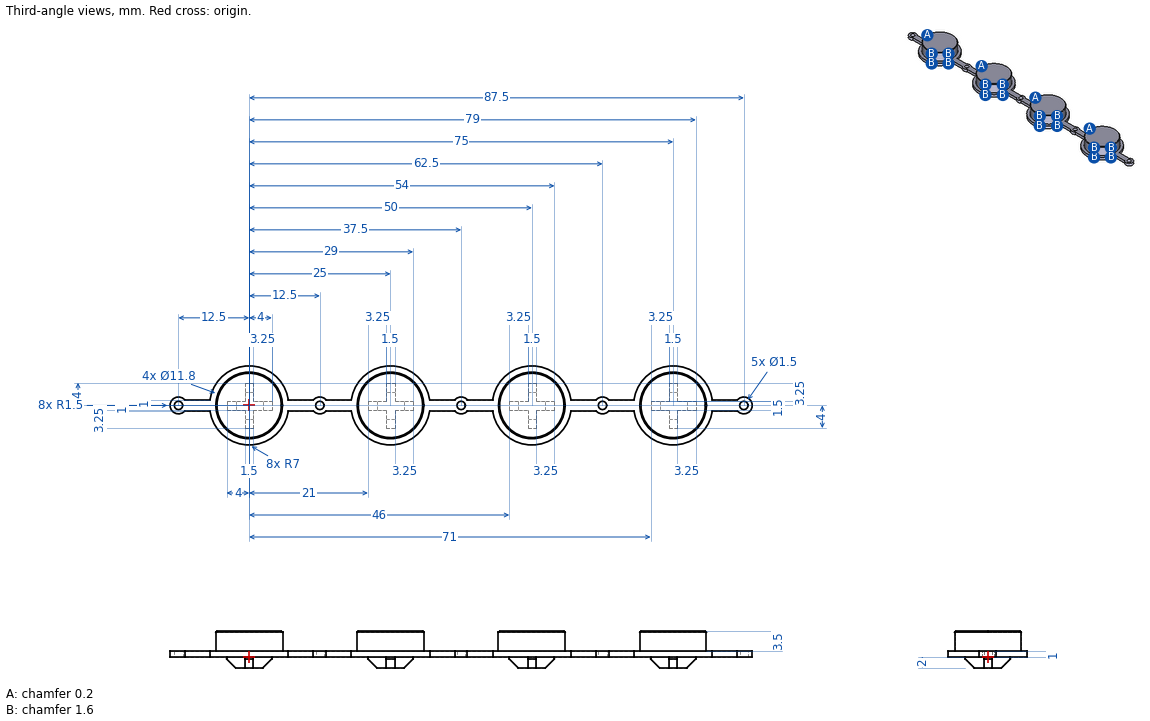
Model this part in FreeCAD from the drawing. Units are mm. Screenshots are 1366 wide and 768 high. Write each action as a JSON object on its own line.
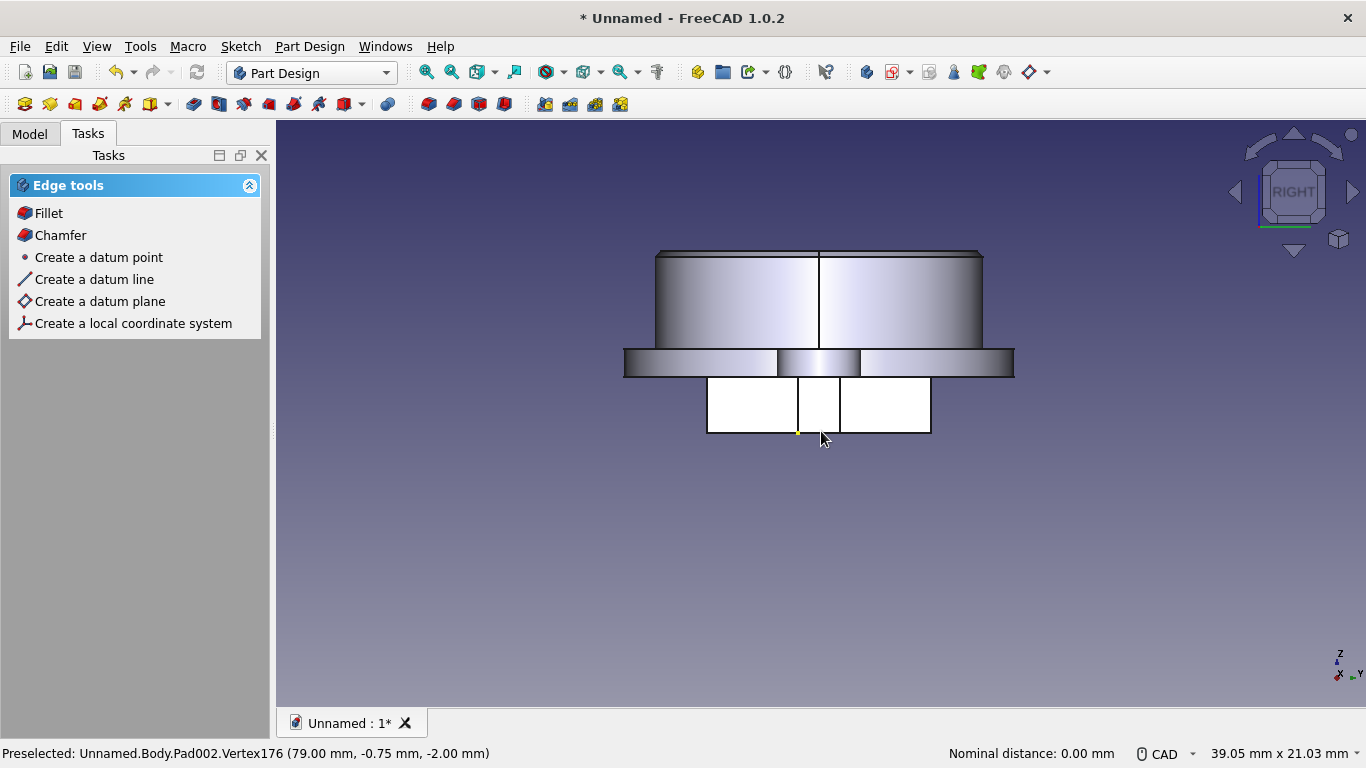
{"action": "left_click", "coordinate": [819, 432], "text": "ctrl"}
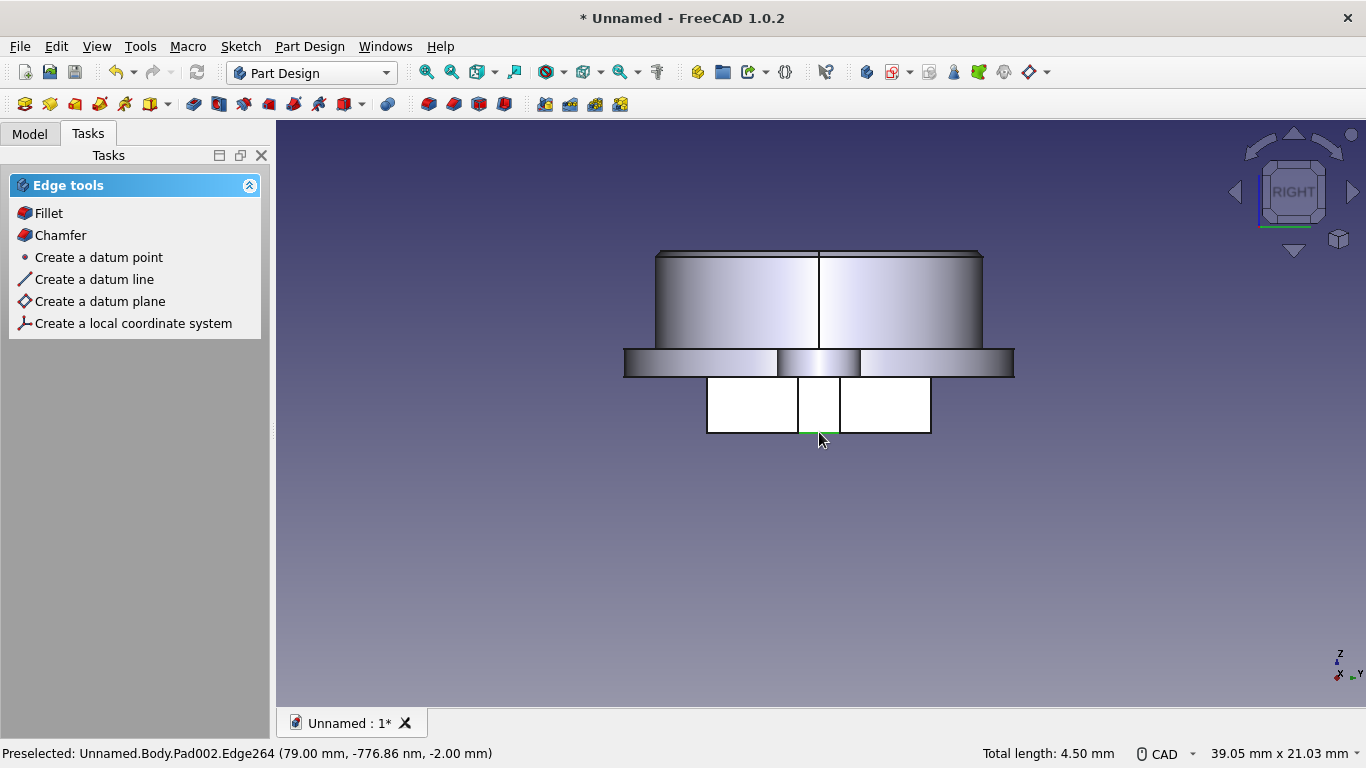
{"action": "key", "text": "v f"}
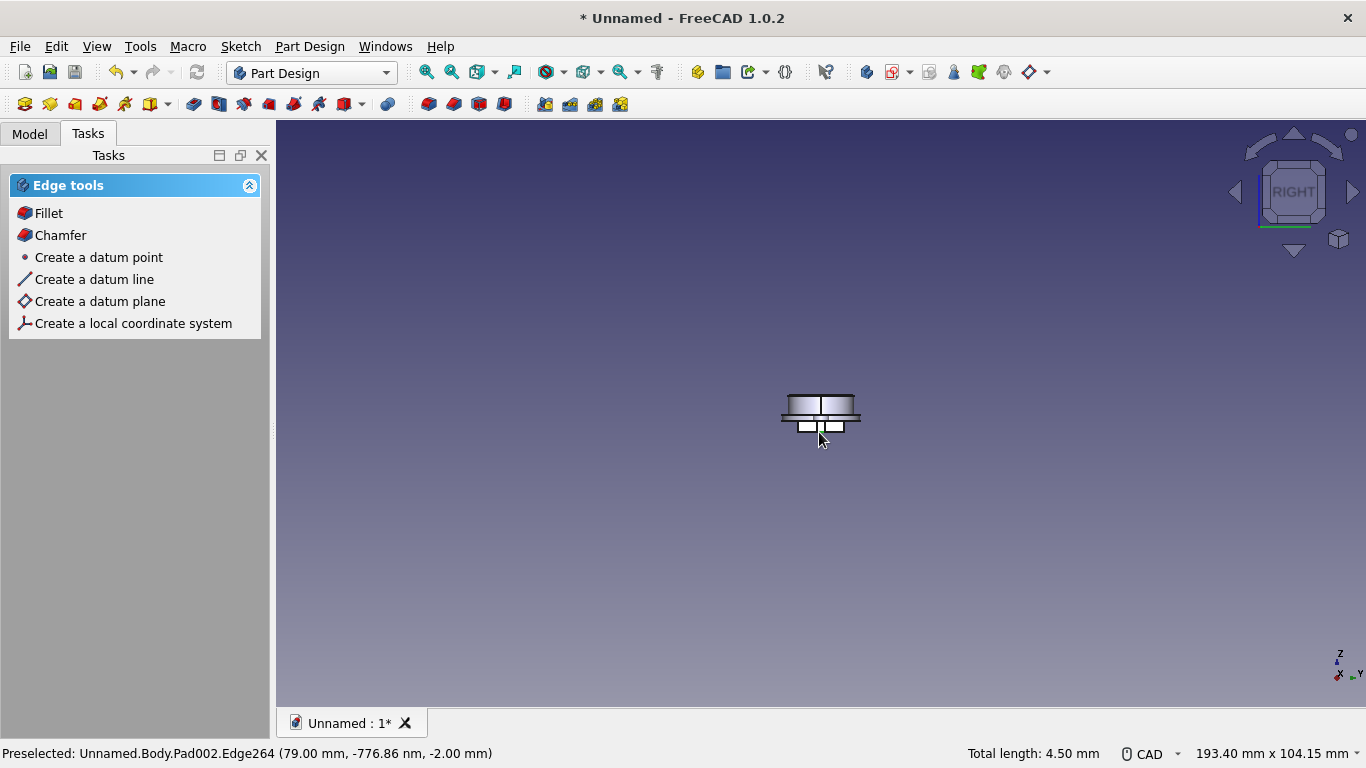
{"action": "key", "text": "5"}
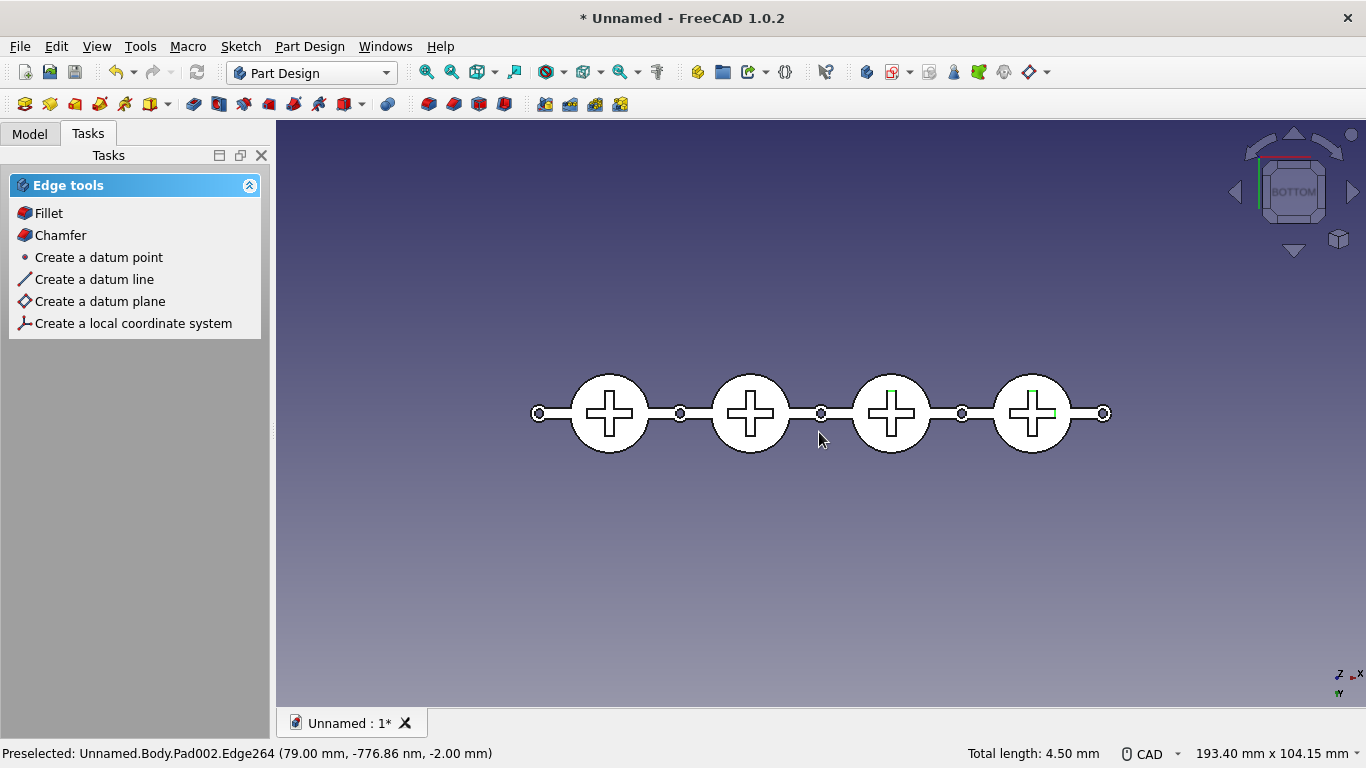
{"action": "scroll", "coordinate": [1010, 412], "scroll_direction": "up", "scroll_amount": 8}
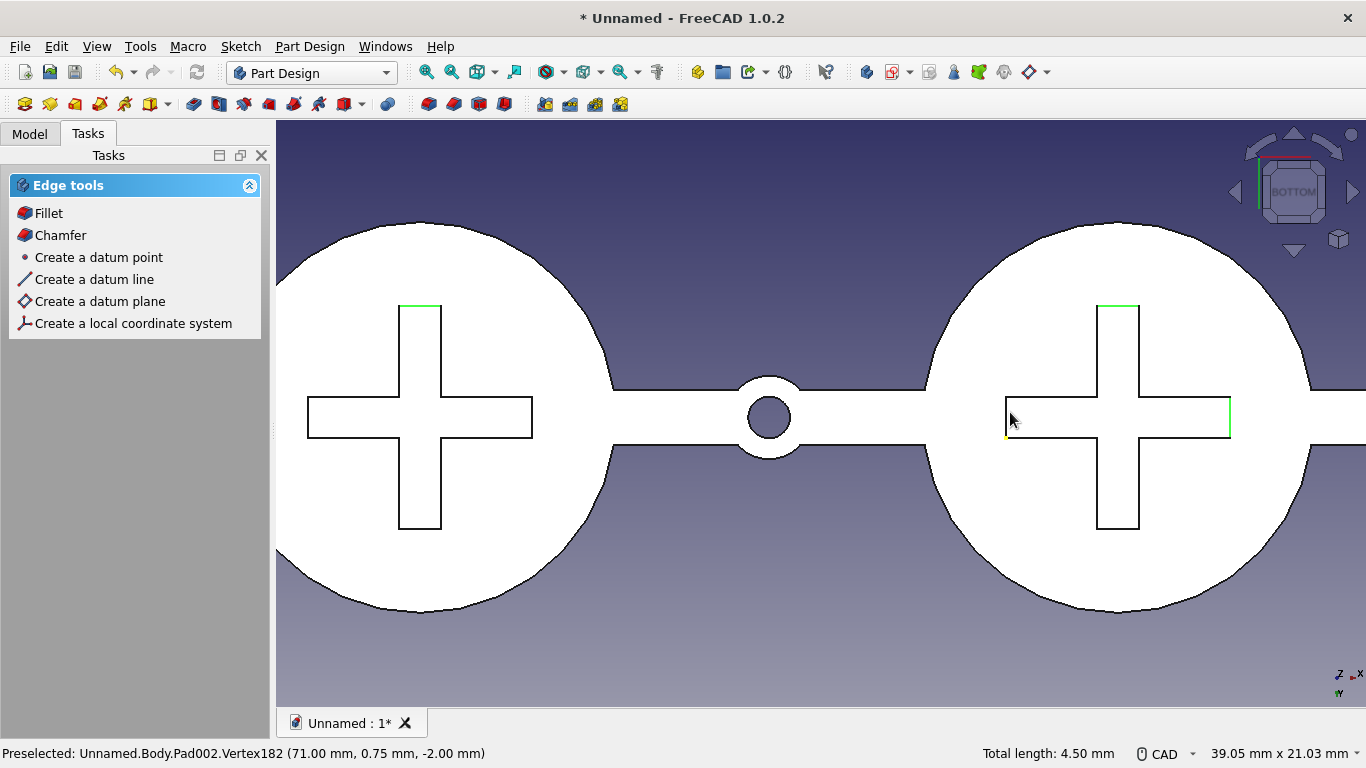
{"action": "left_click", "coordinate": [1006, 416], "text": "ctrl"}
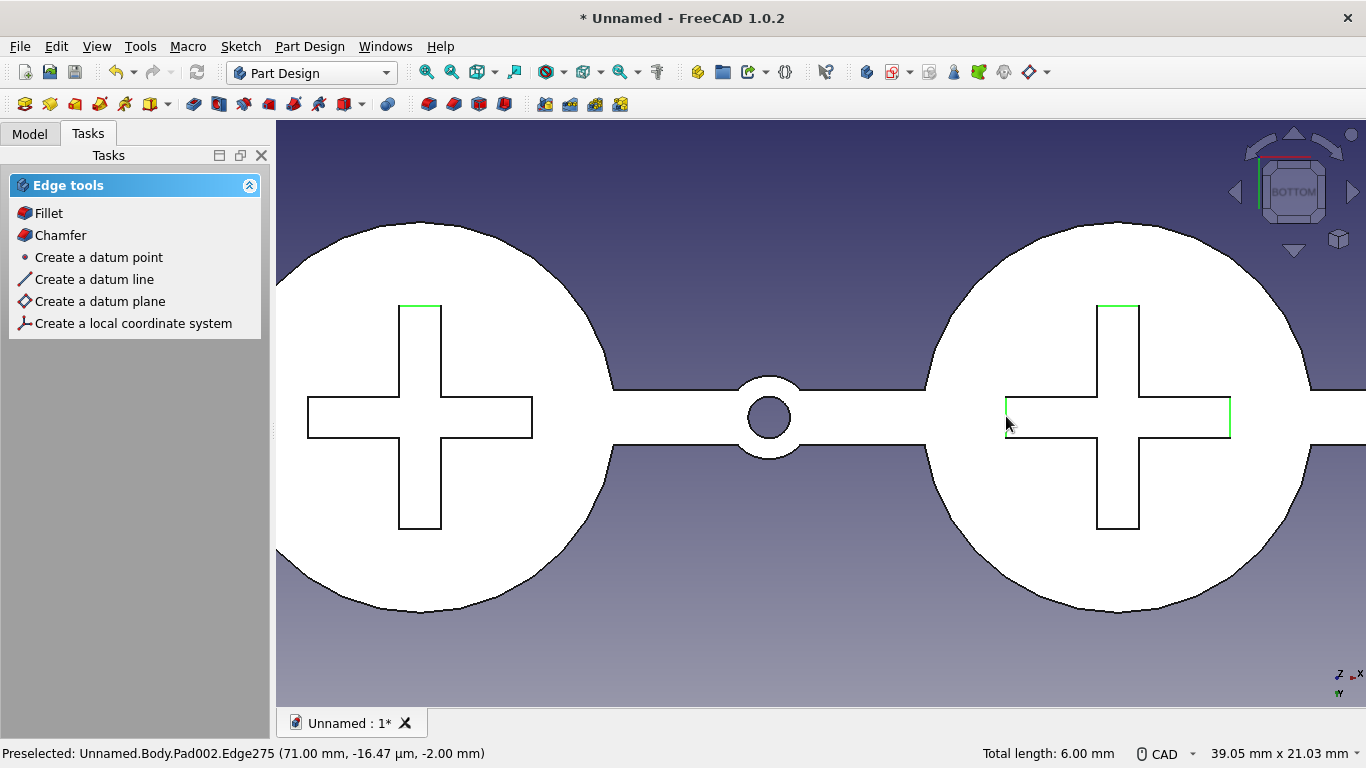
{"action": "left_click", "coordinate": [1118, 528], "text": "ctrl"}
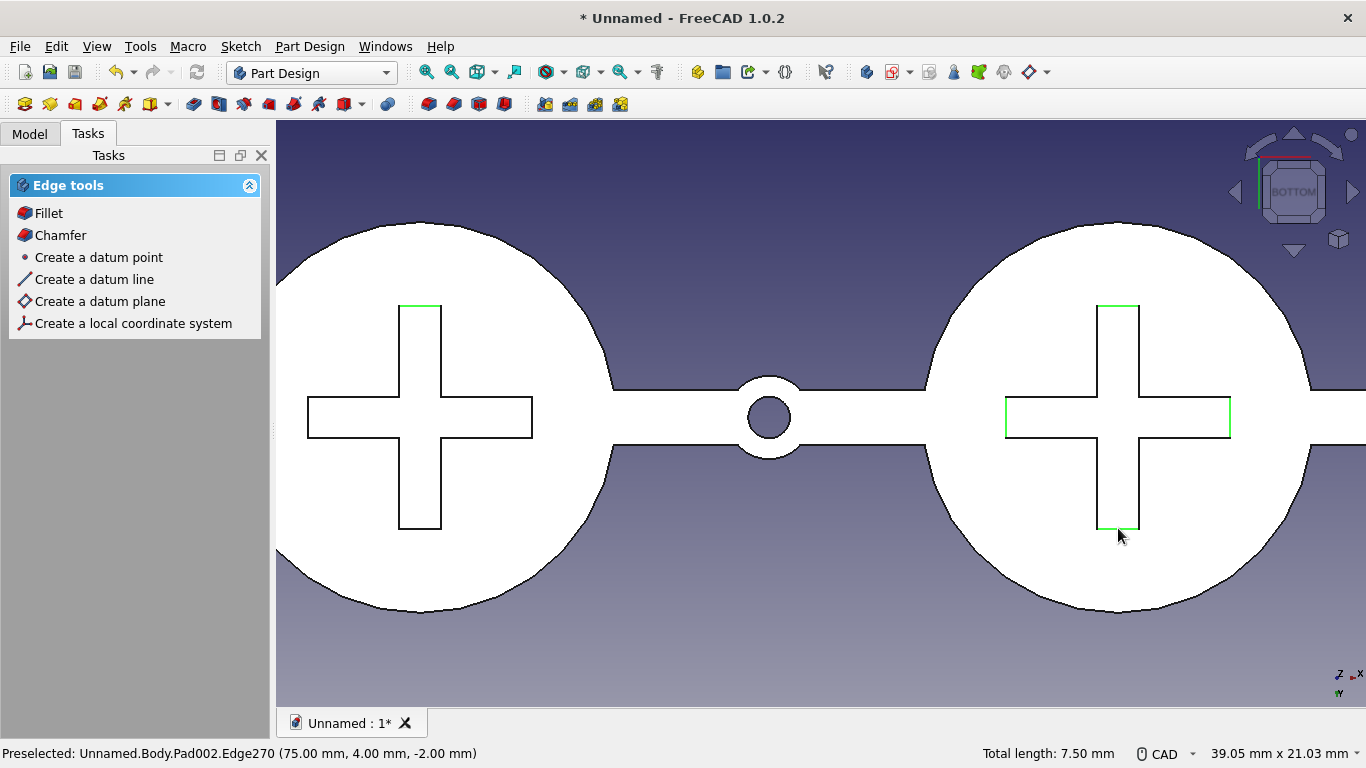
{"action": "left_click", "coordinate": [308, 416], "text": "ctrl"}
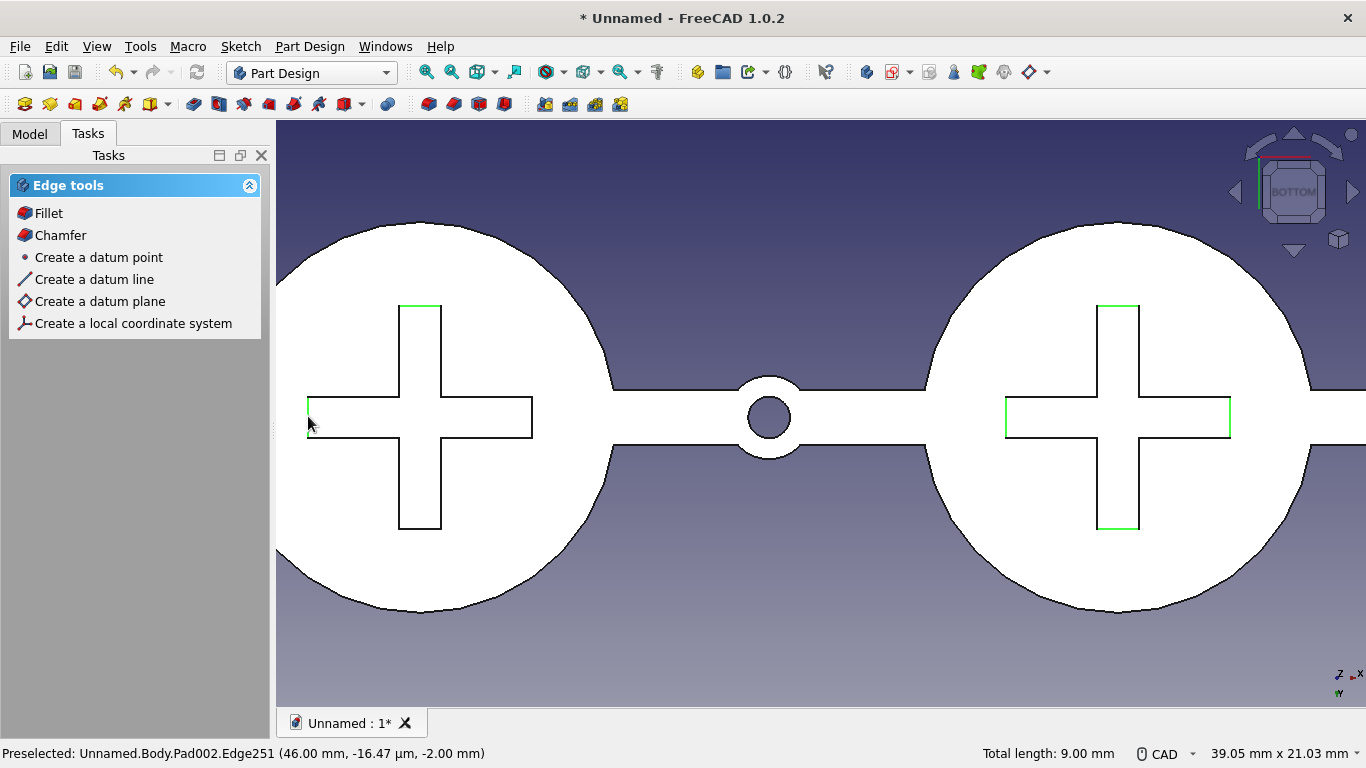
{"action": "left_click", "coordinate": [420, 528], "text": "ctrl"}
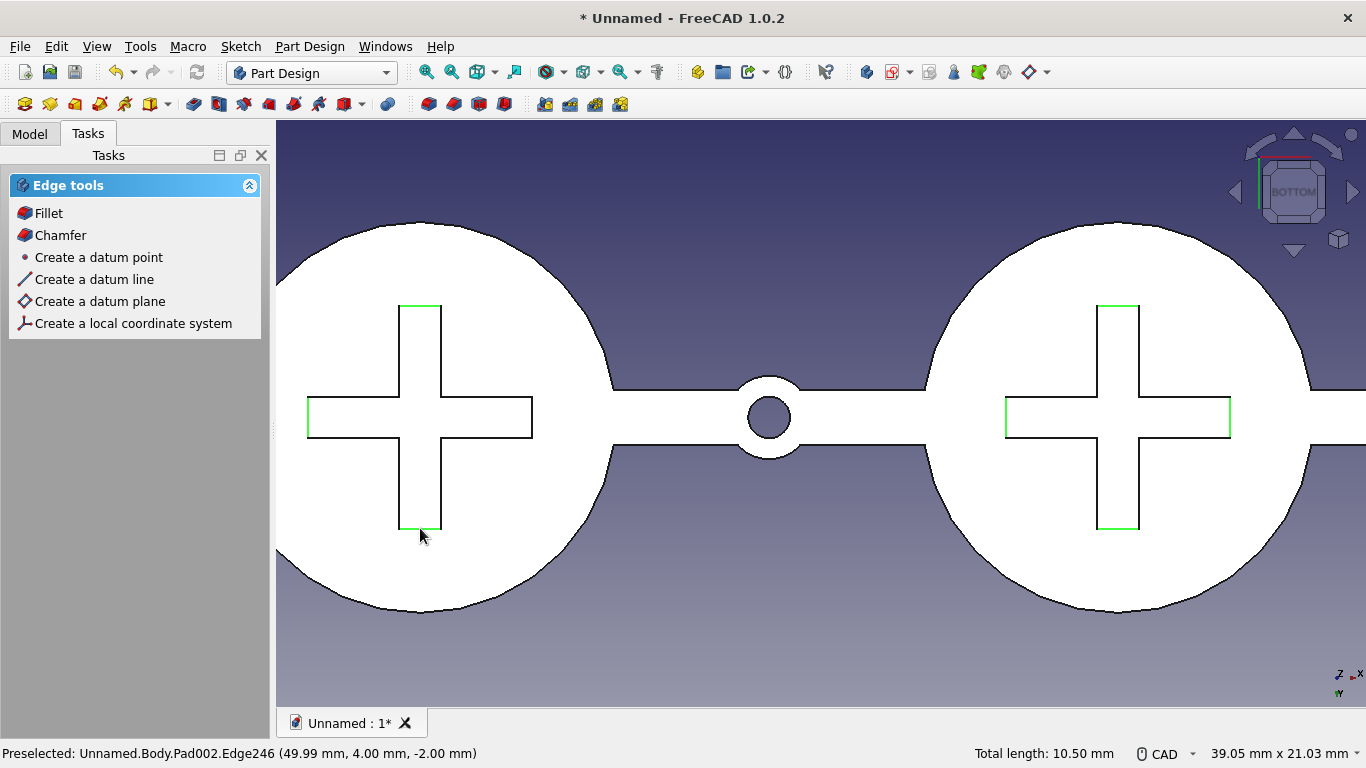
{"action": "left_click", "coordinate": [532, 416], "text": "ctrl"}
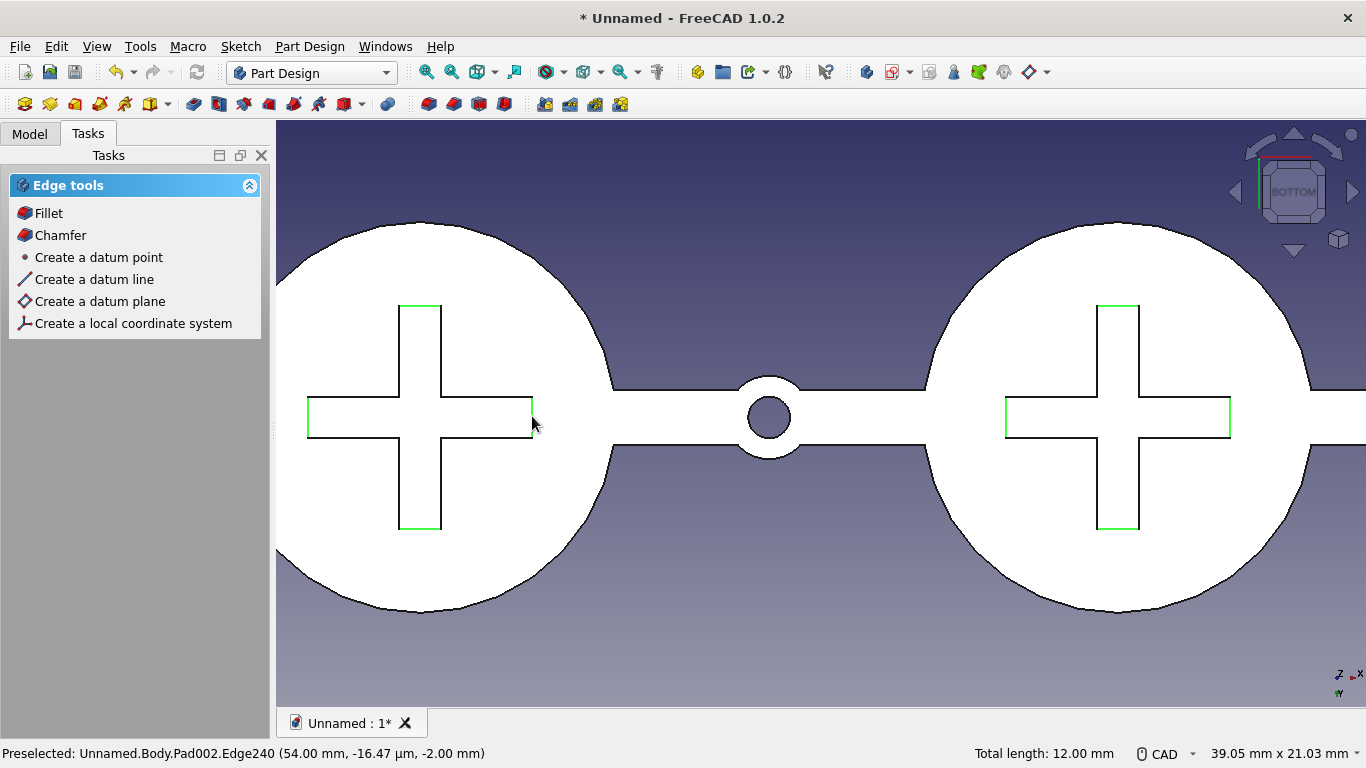
{"action": "left_click", "coordinate": [427, 72]}